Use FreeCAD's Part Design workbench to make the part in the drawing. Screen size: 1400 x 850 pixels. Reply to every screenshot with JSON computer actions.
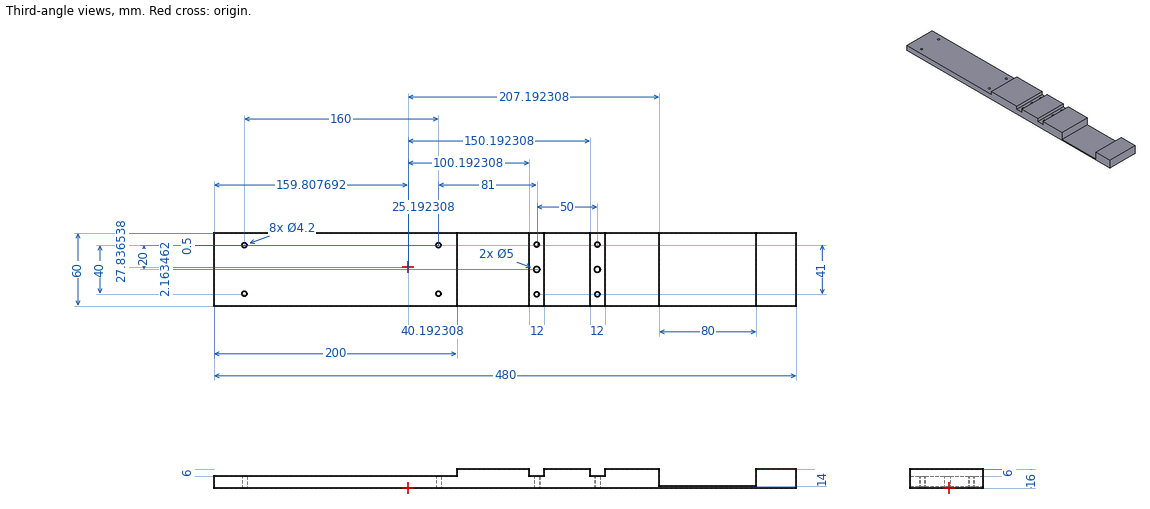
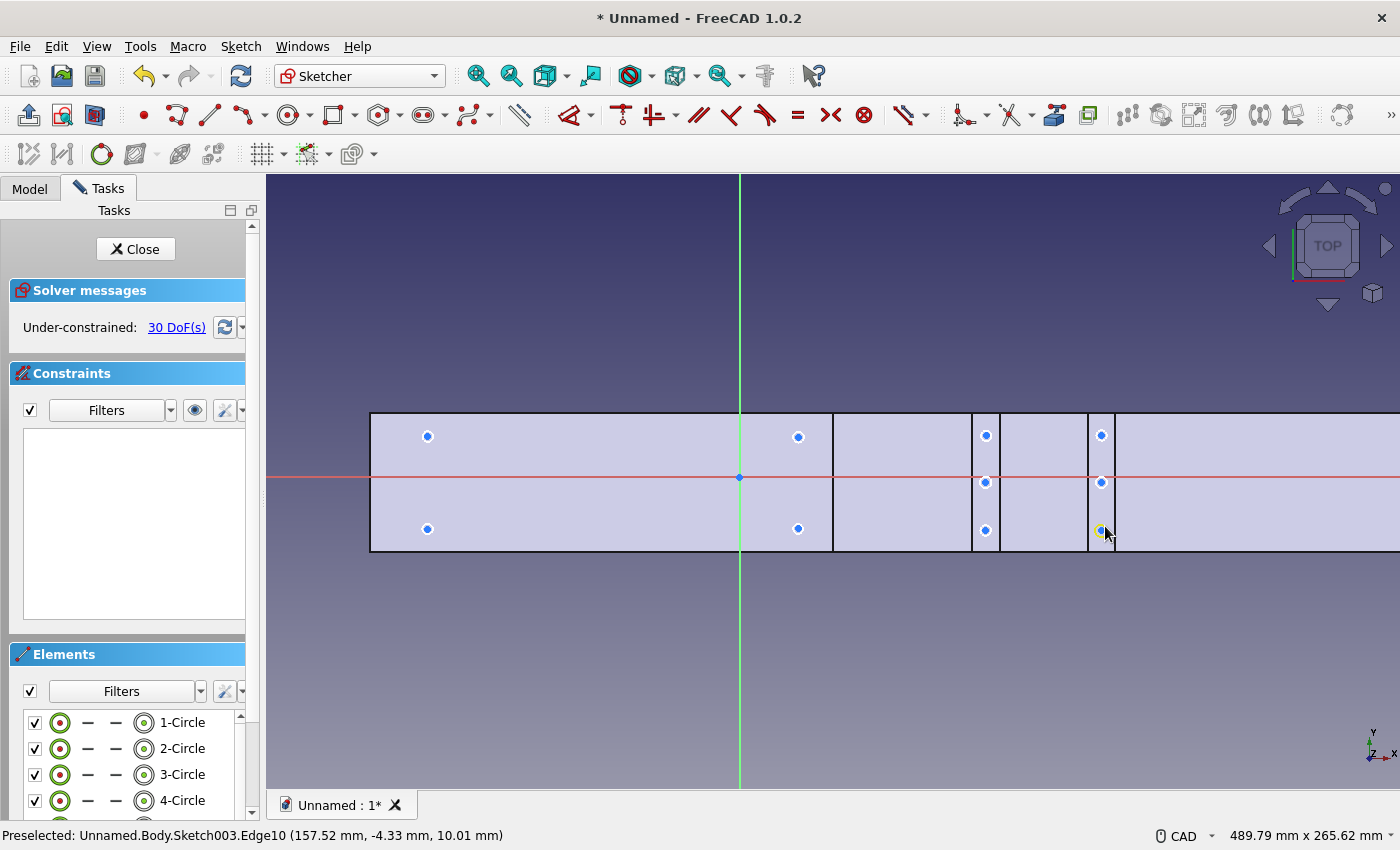
{"action": "scroll", "coordinate": [431, 433], "scroll_direction": "up", "scroll_amount": 5}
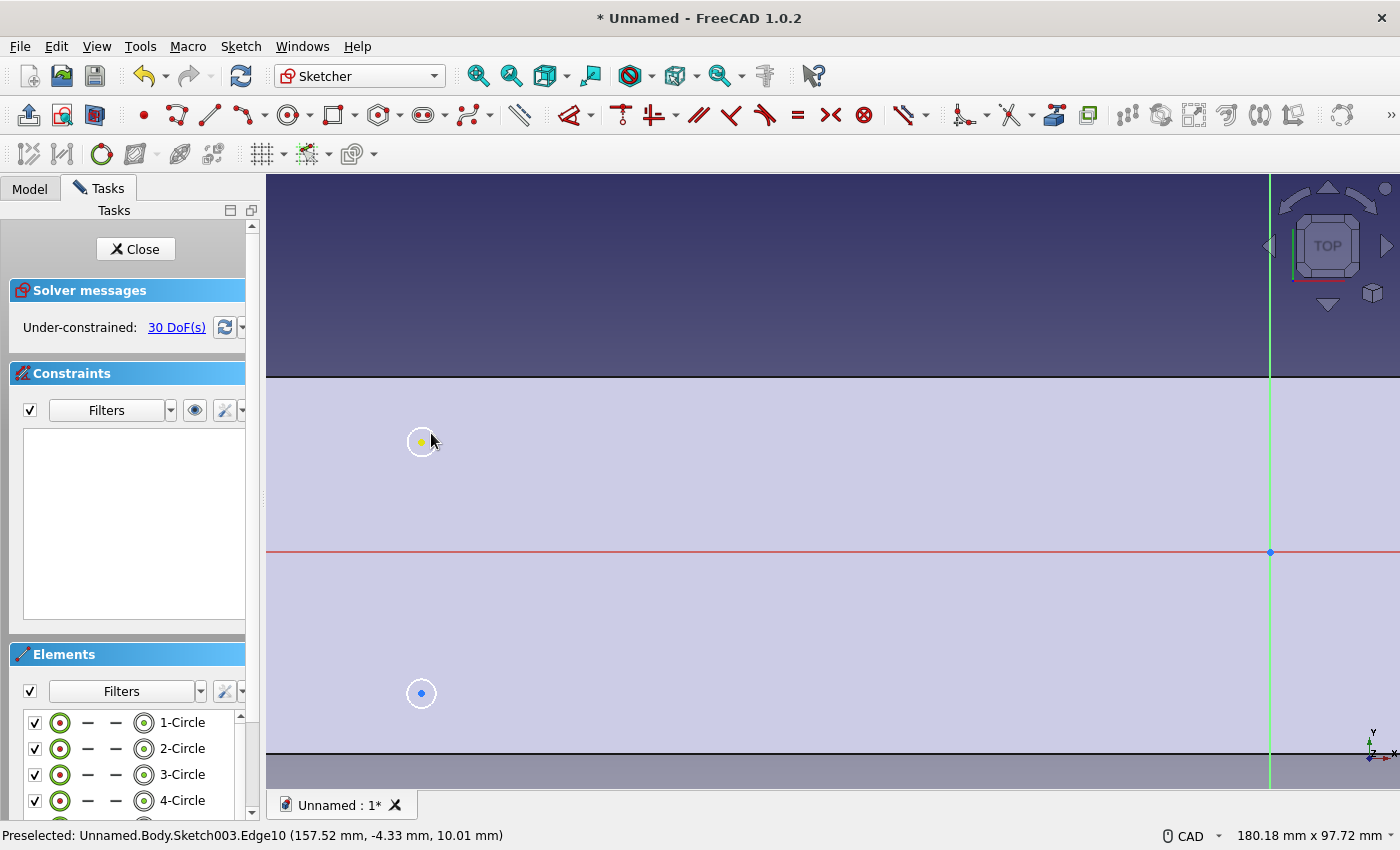
{"action": "left_click", "coordinate": [432, 432]}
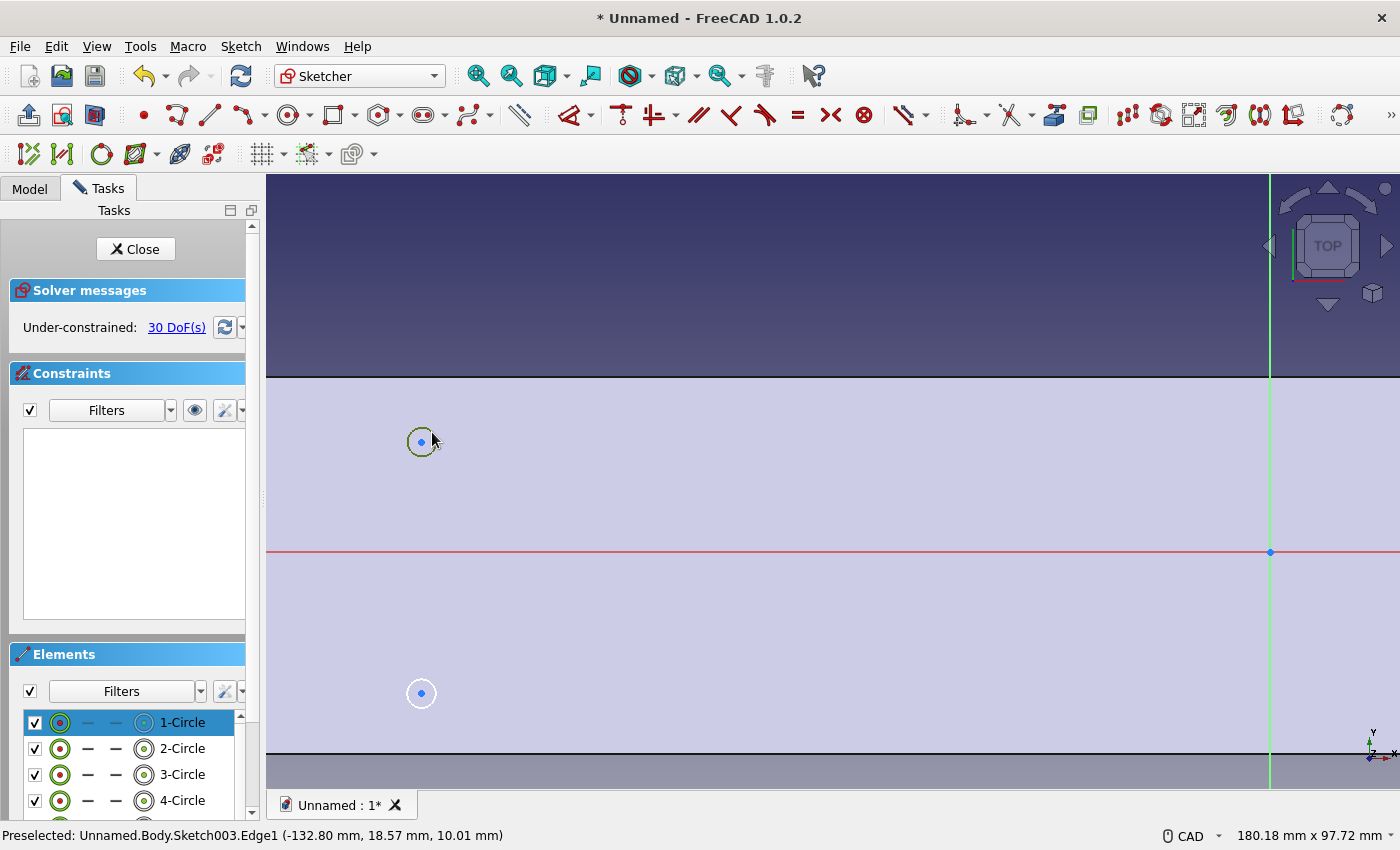
{"action": "left_click", "coordinate": [432, 684]}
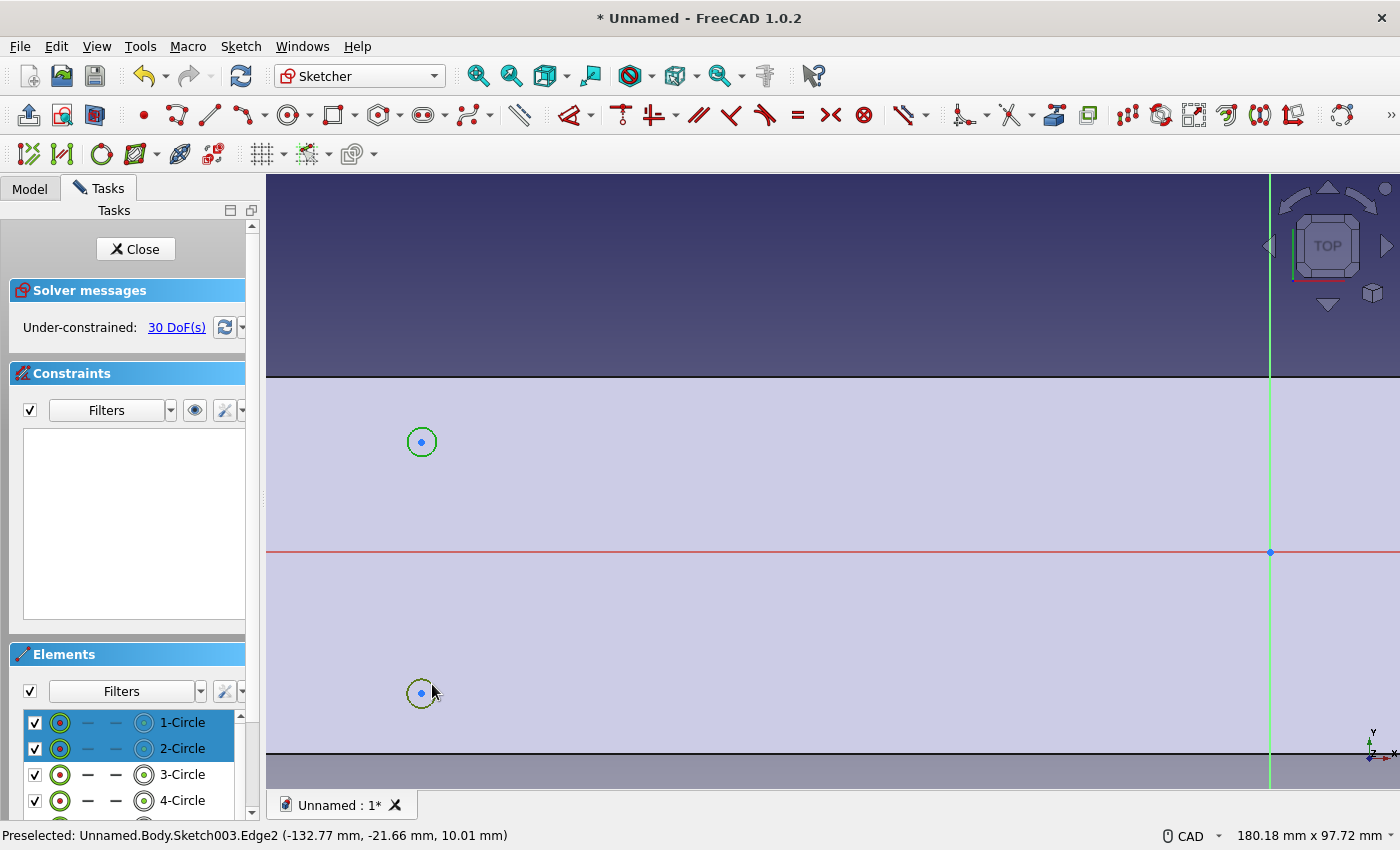
{"action": "scroll", "coordinate": [430, 433], "scroll_direction": "down", "scroll_amount": 5}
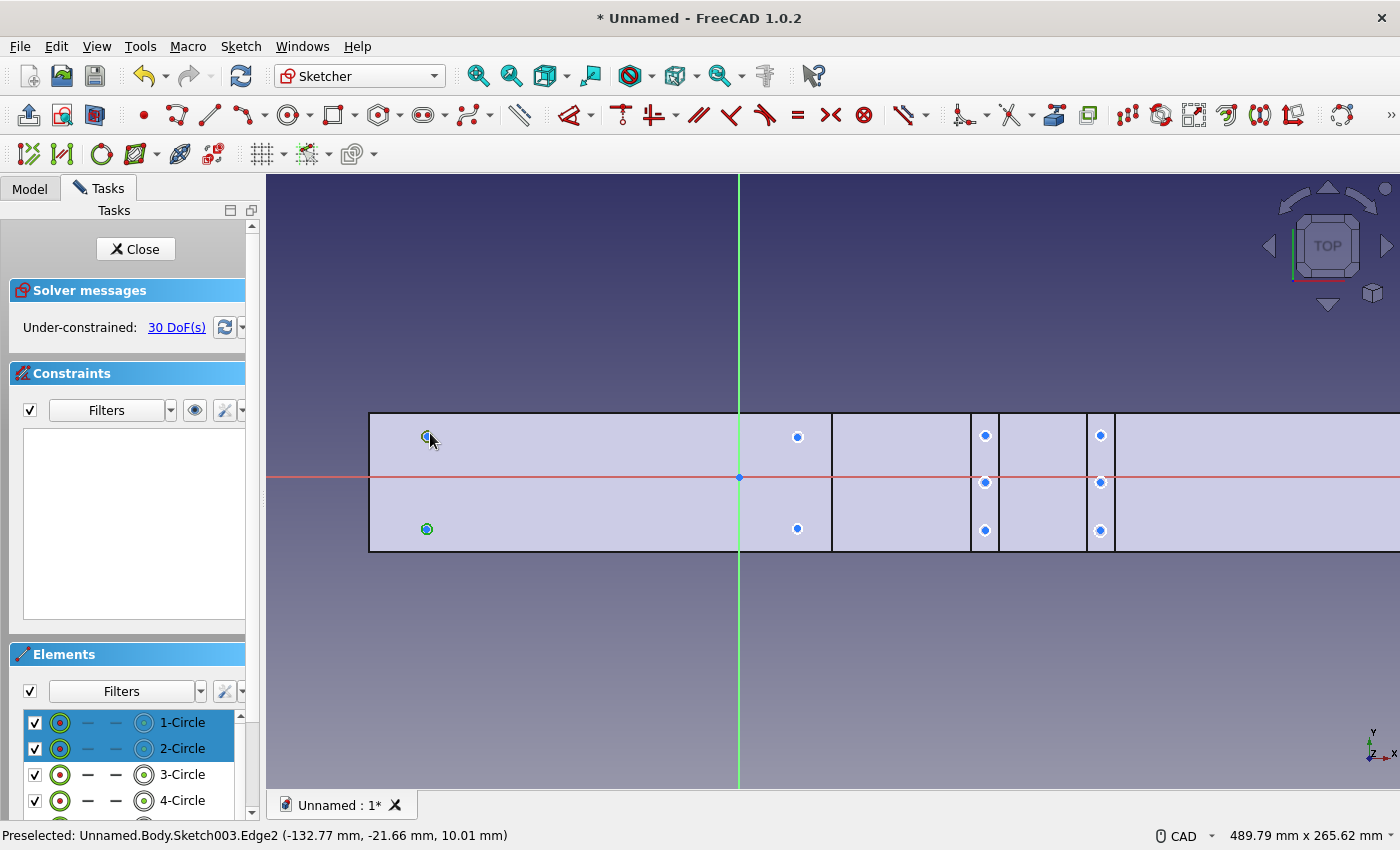
{"action": "scroll", "coordinate": [802, 433], "scroll_direction": "up", "scroll_amount": 5}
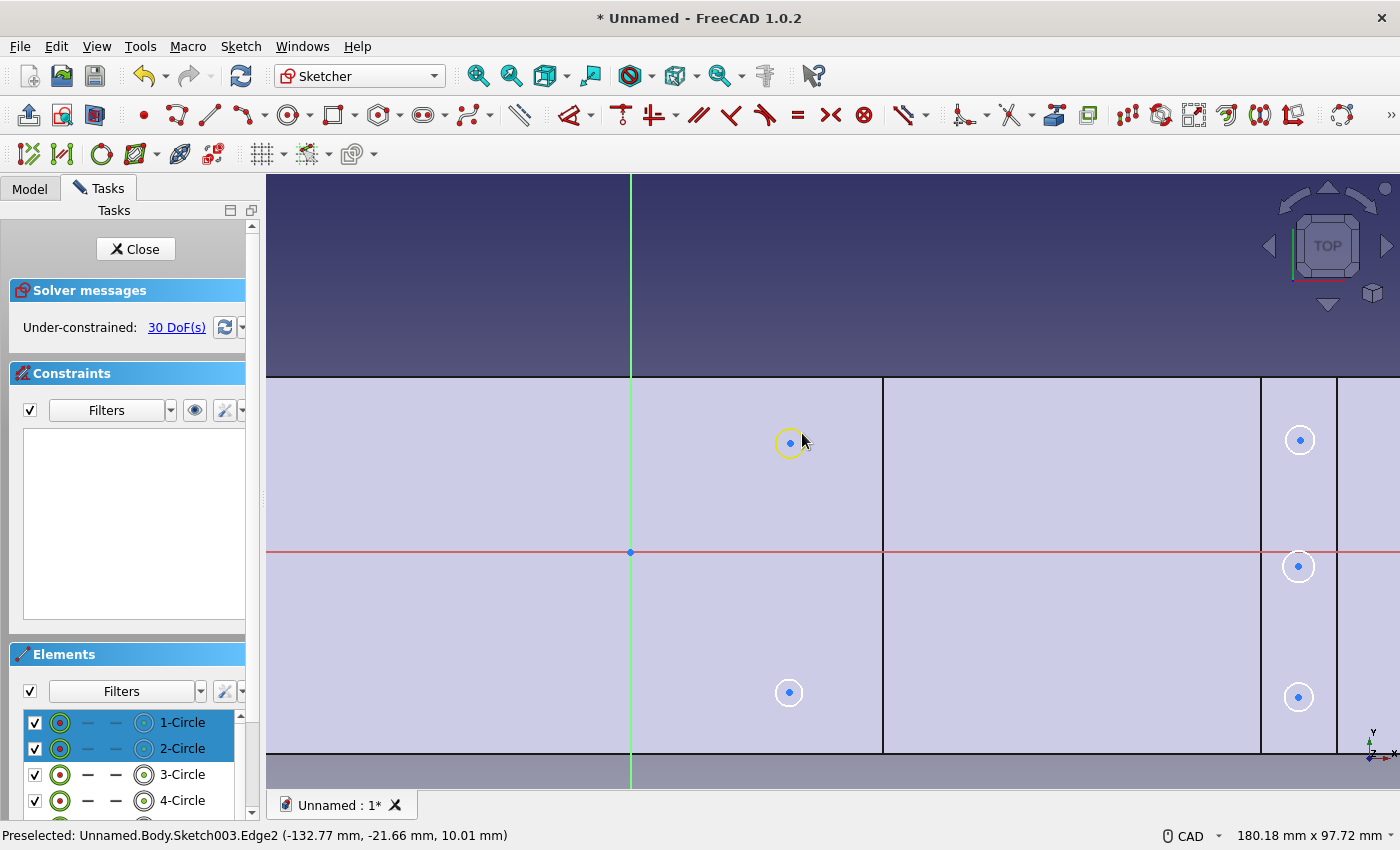
{"action": "left_click", "coordinate": [800, 433]}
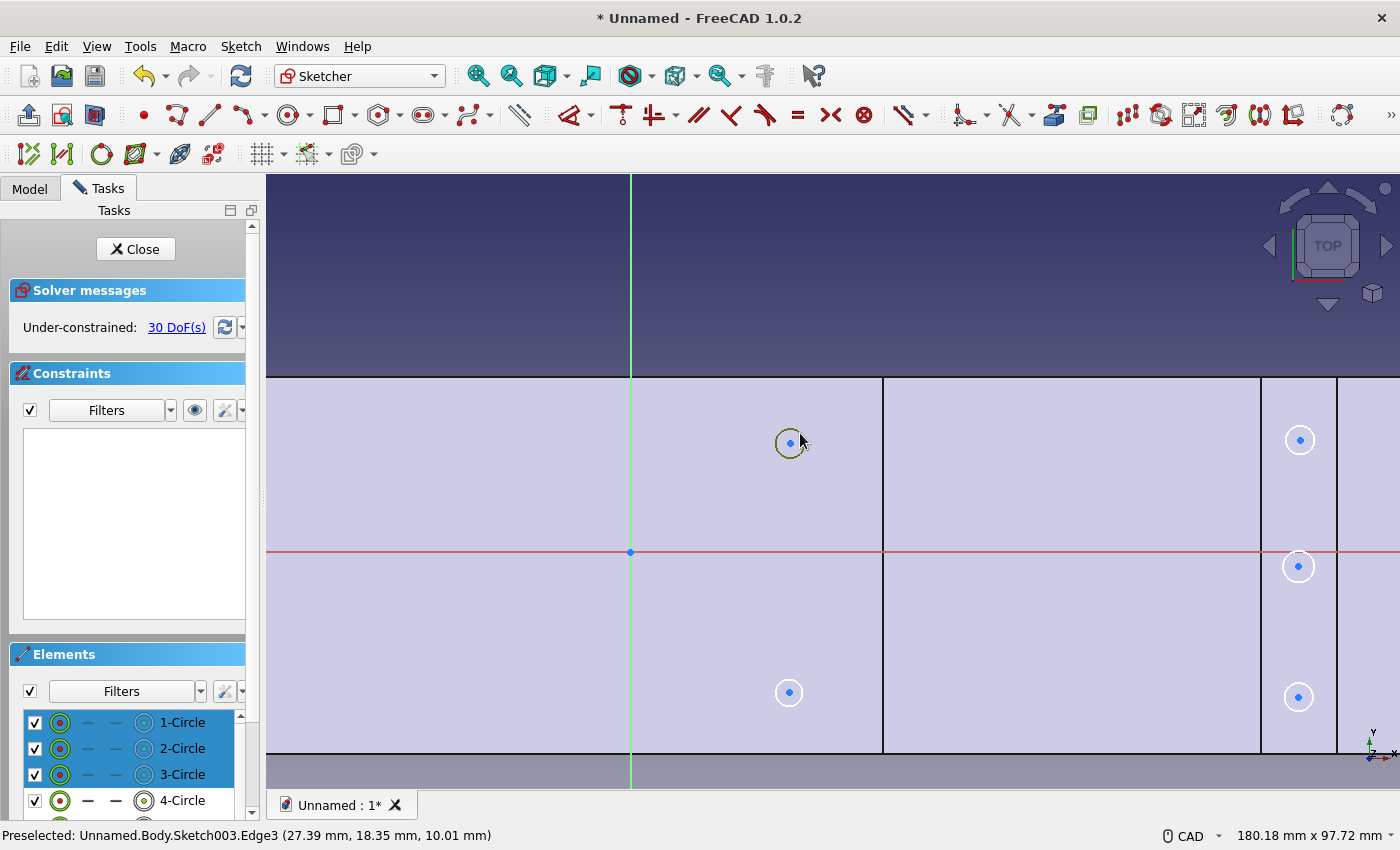
{"action": "left_click", "coordinate": [799, 684]}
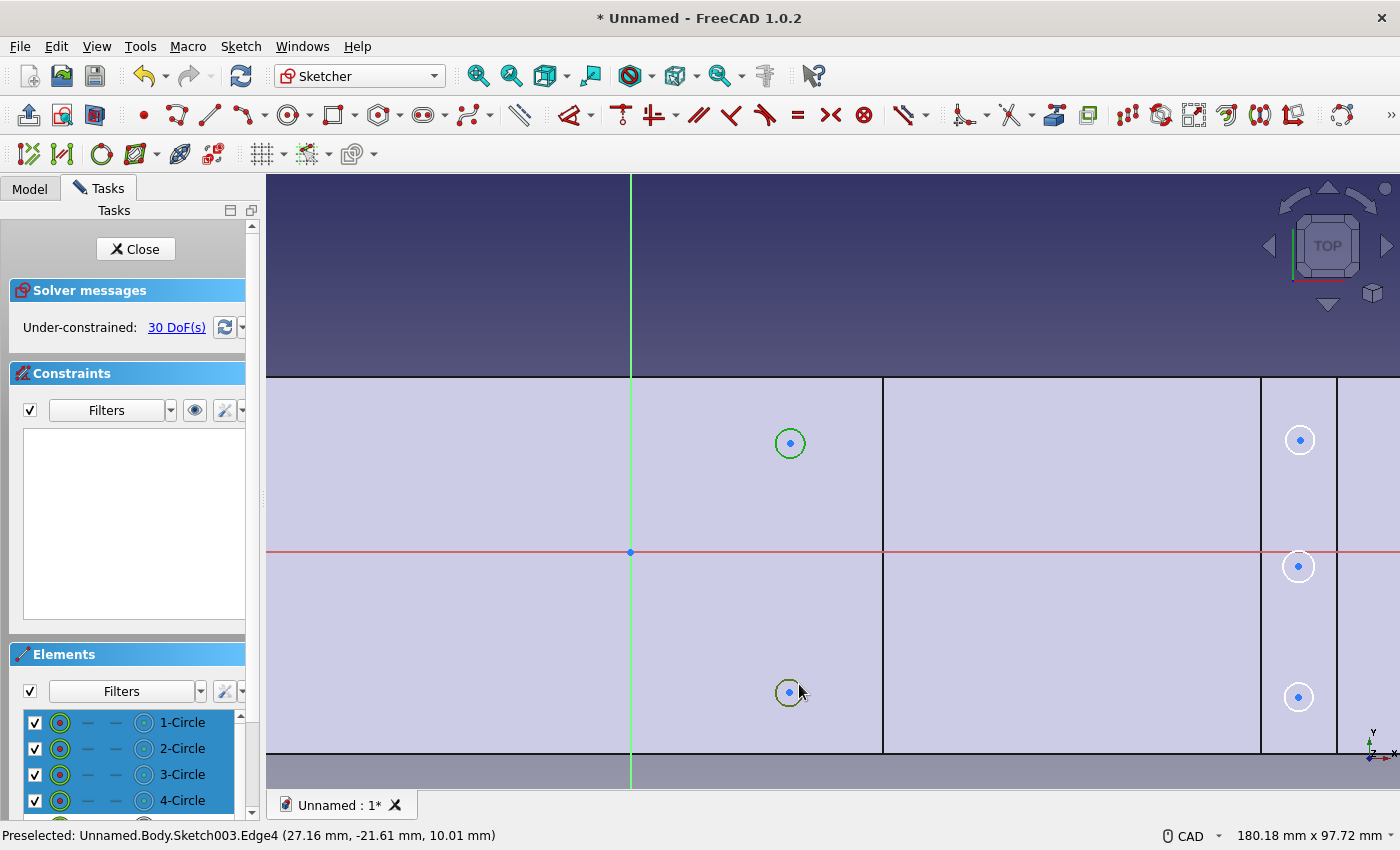
{"action": "scroll", "coordinate": [803, 433], "scroll_direction": "down", "scroll_amount": 5}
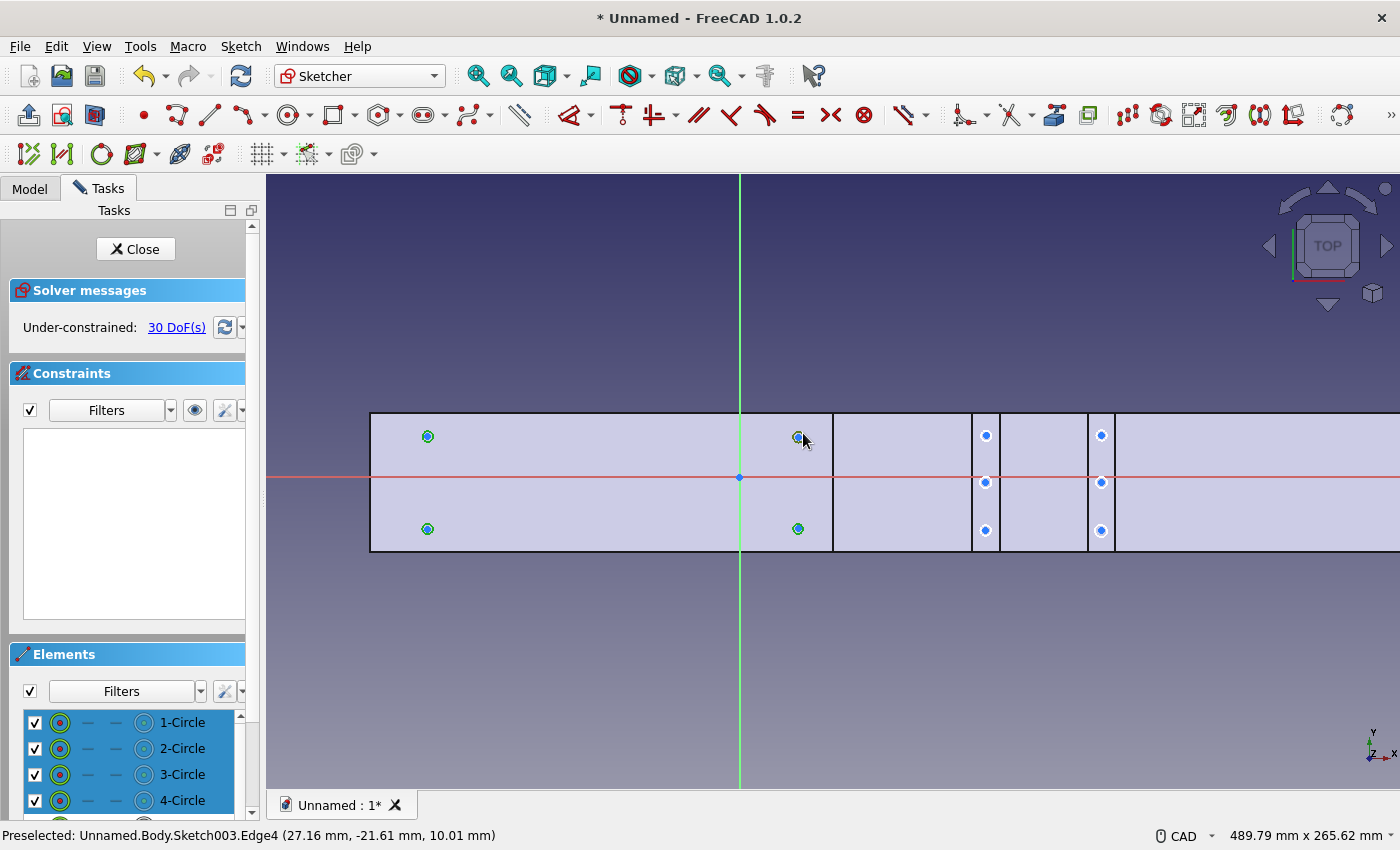
{"action": "scroll", "coordinate": [990, 432], "scroll_direction": "up", "scroll_amount": 5}